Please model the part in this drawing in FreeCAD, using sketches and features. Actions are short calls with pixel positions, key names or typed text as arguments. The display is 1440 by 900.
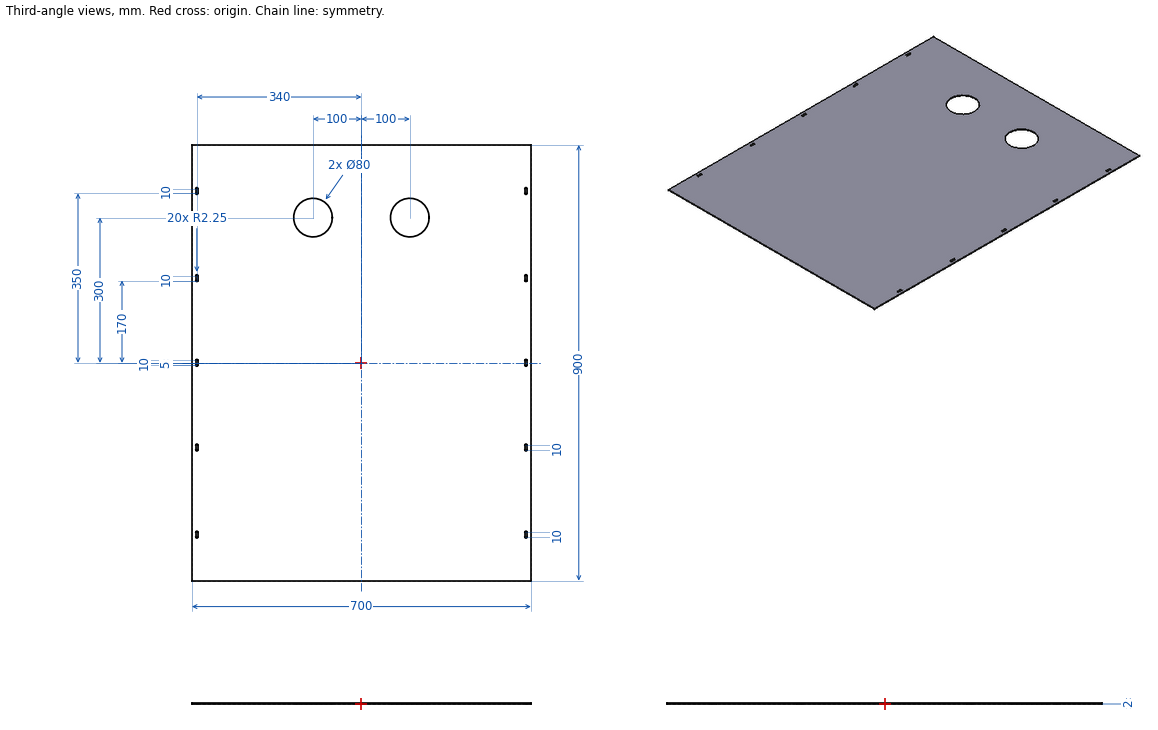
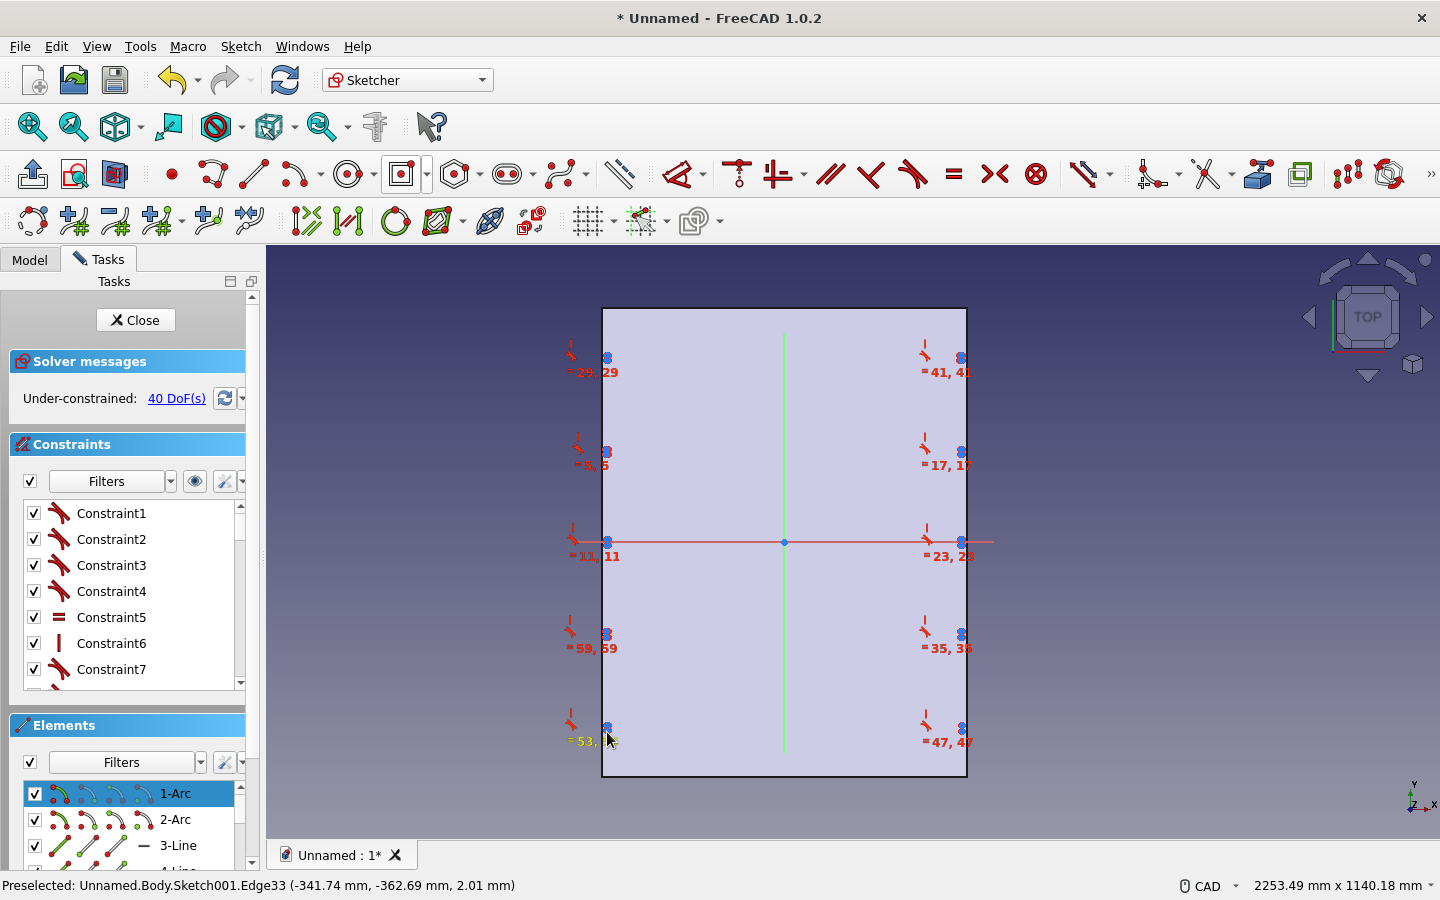
scroll(606, 639, up, 12)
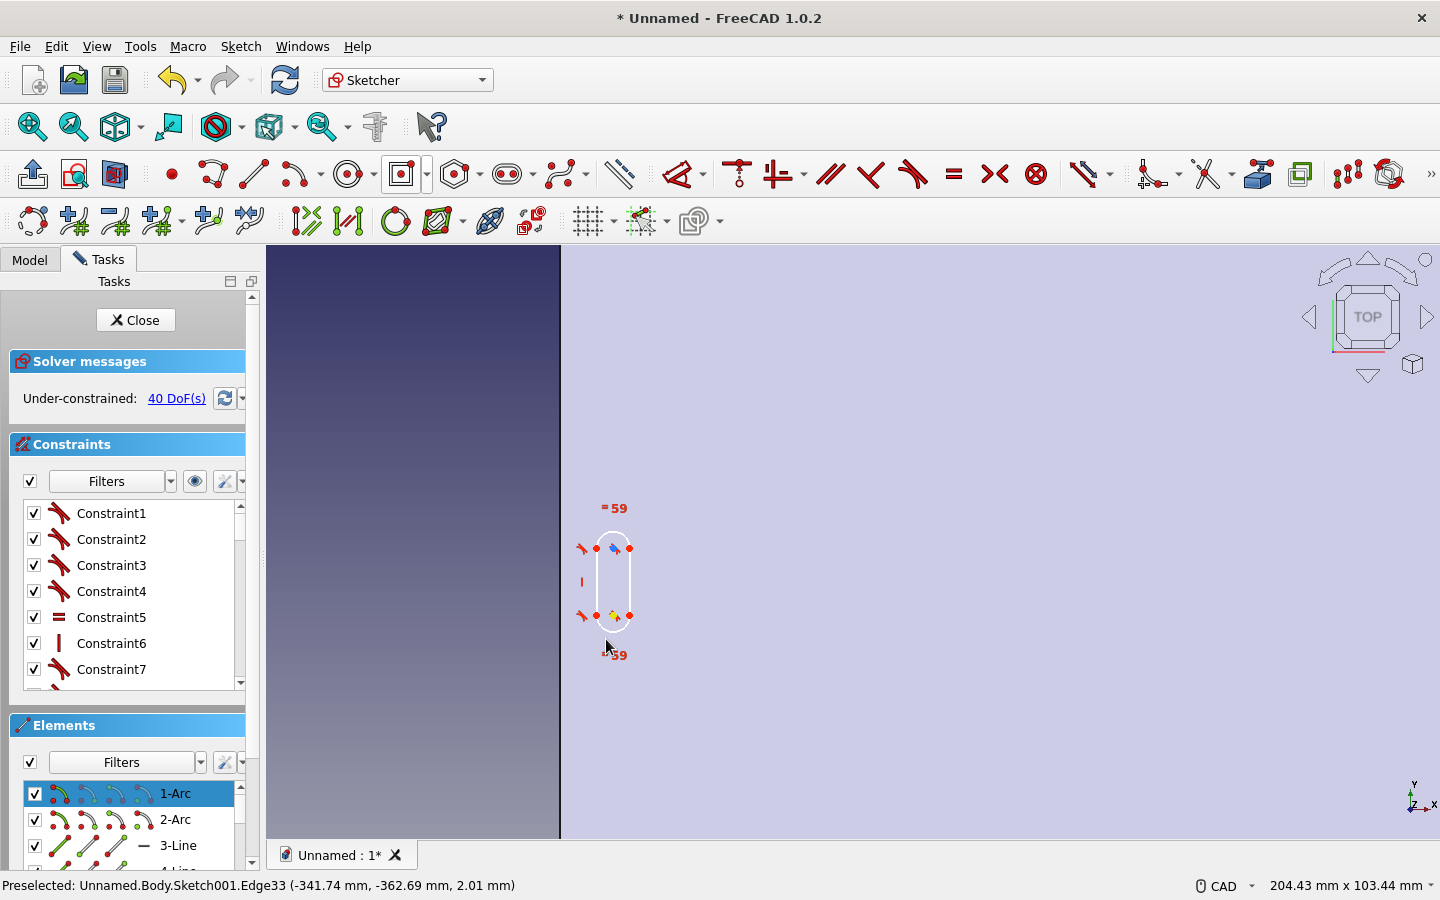
click(604, 629)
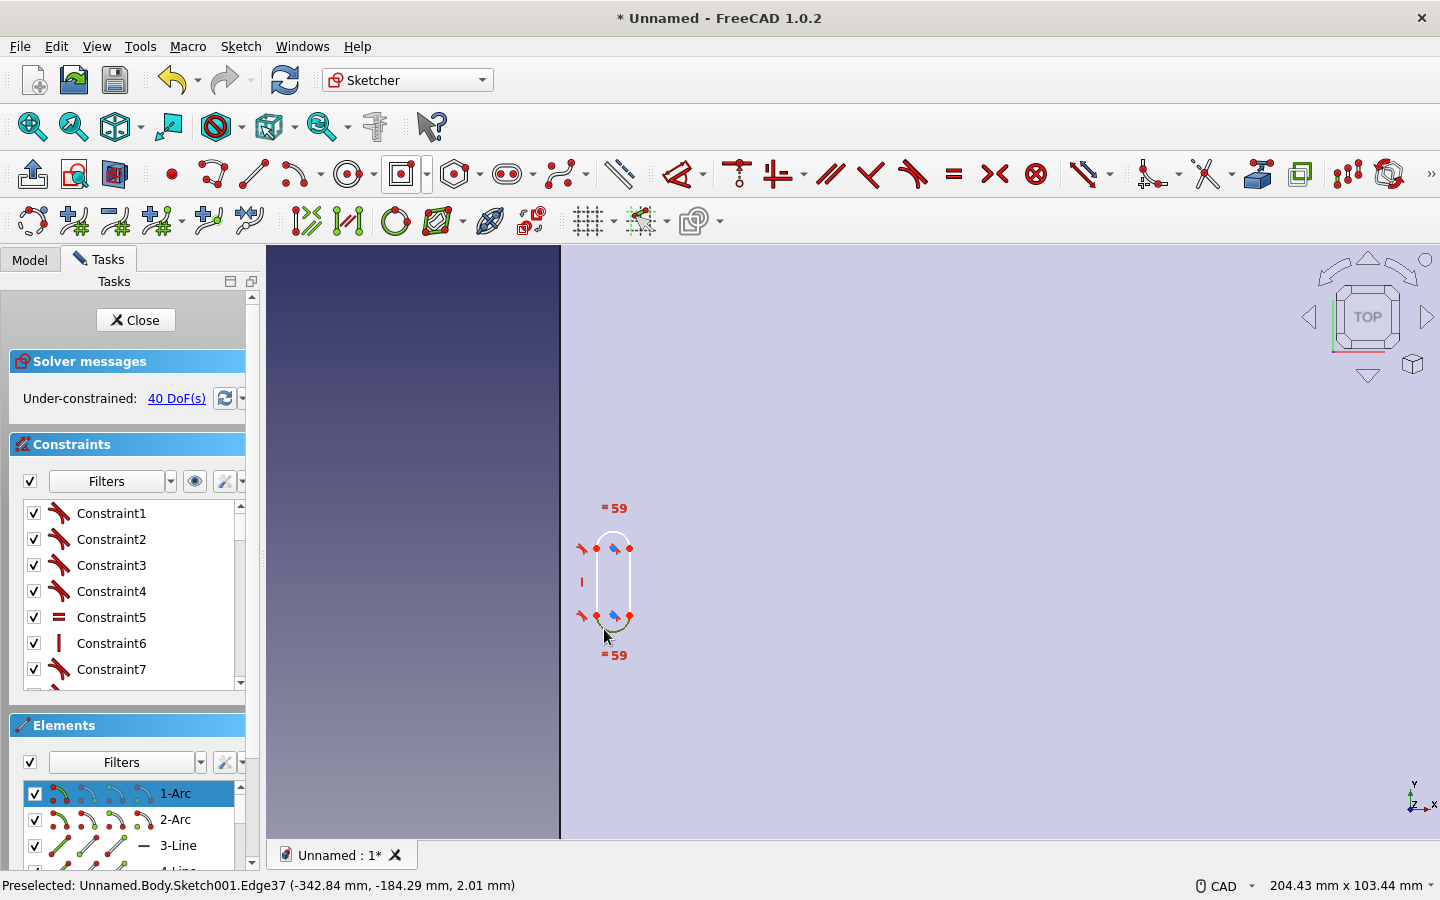
key(e)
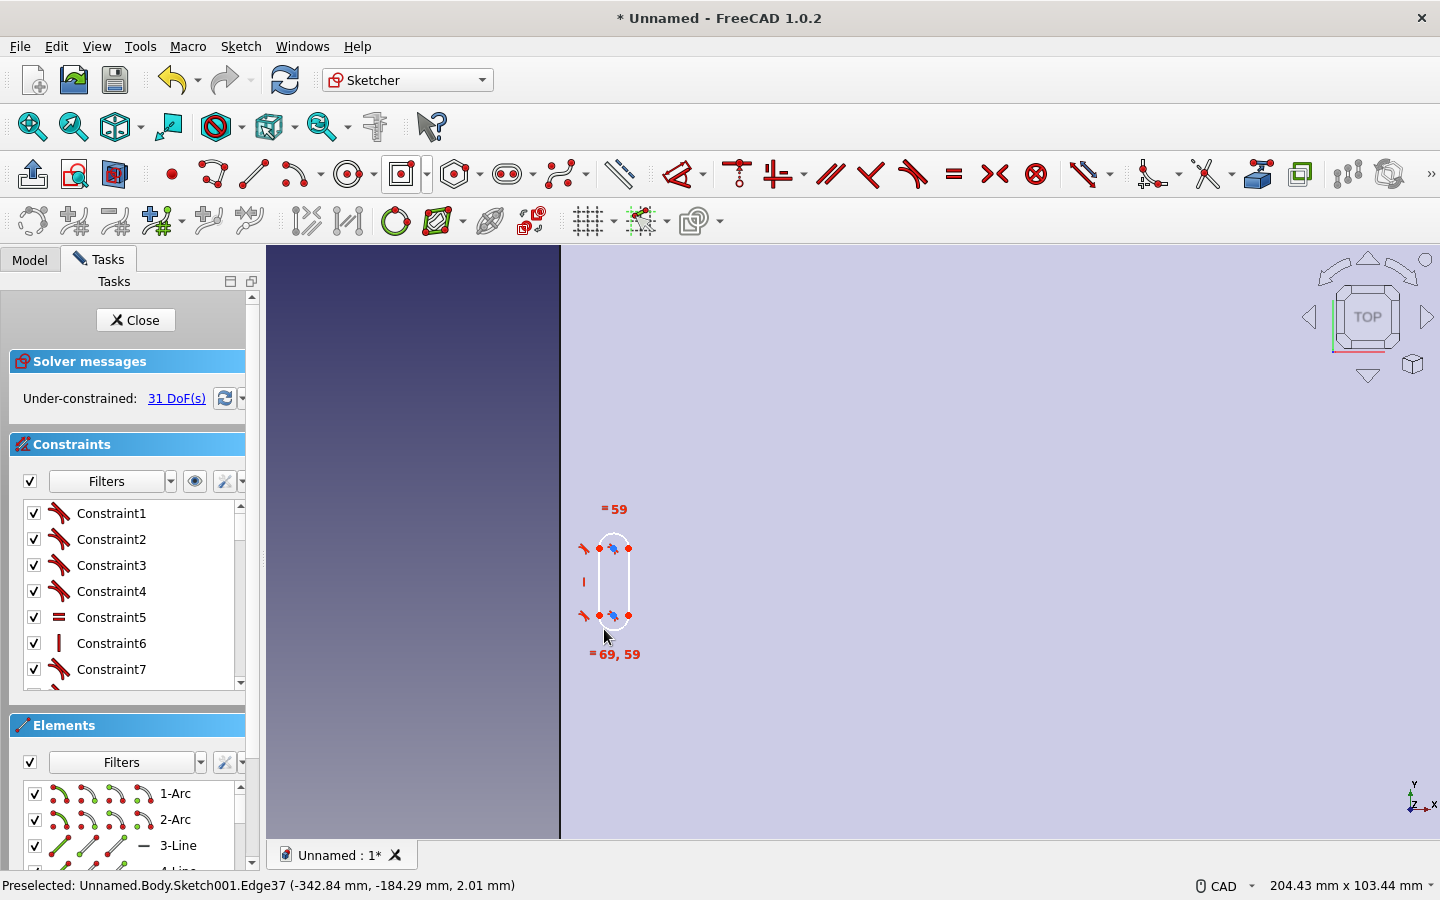
scroll(606, 639, down, 12)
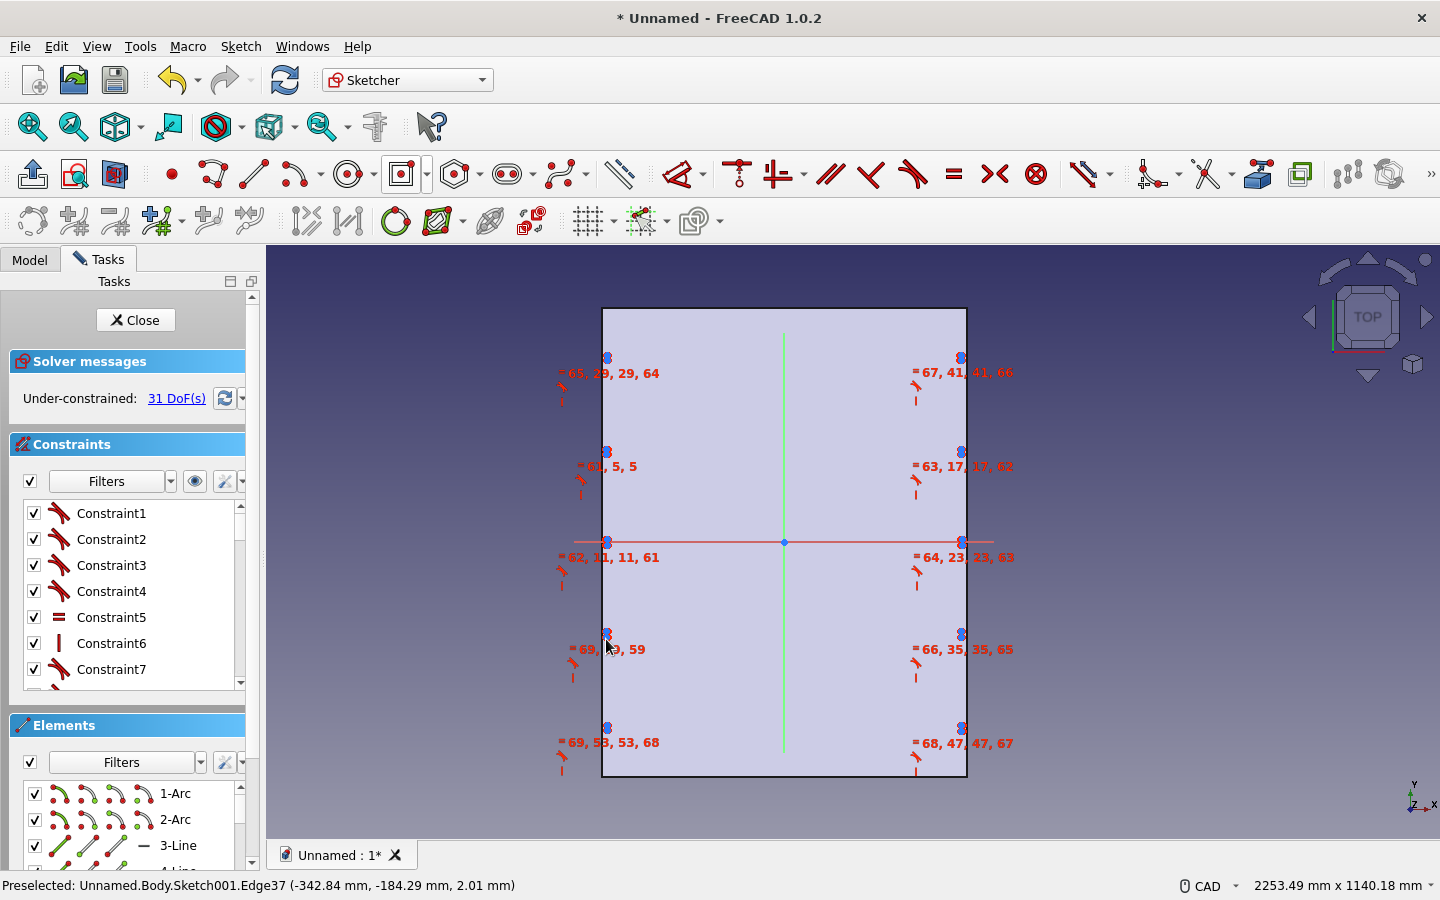
scroll(607, 454, up, 12)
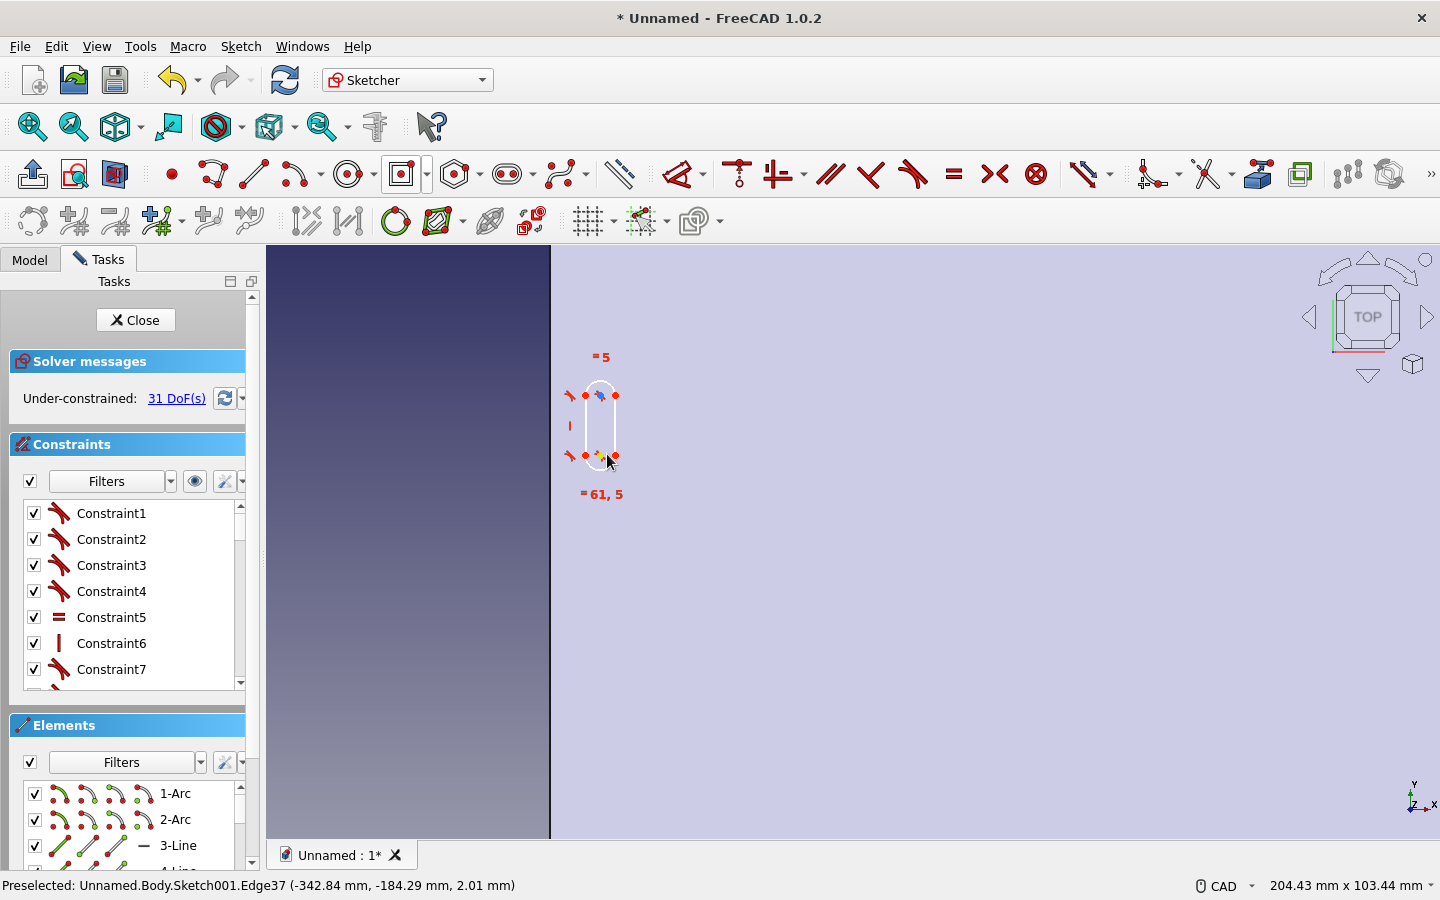
click(600, 456)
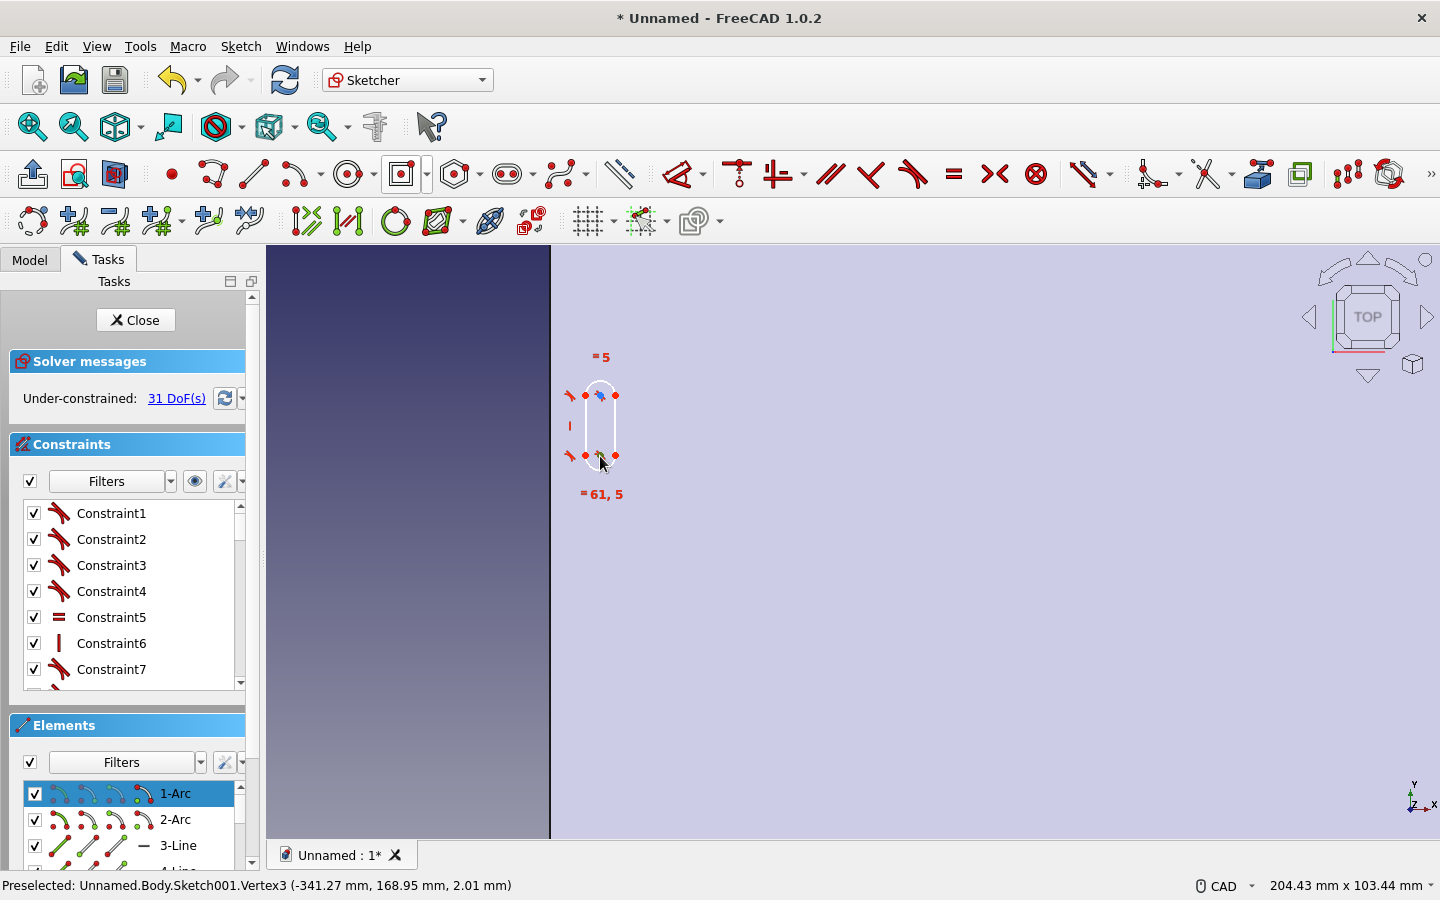
scroll(607, 454, down, 12)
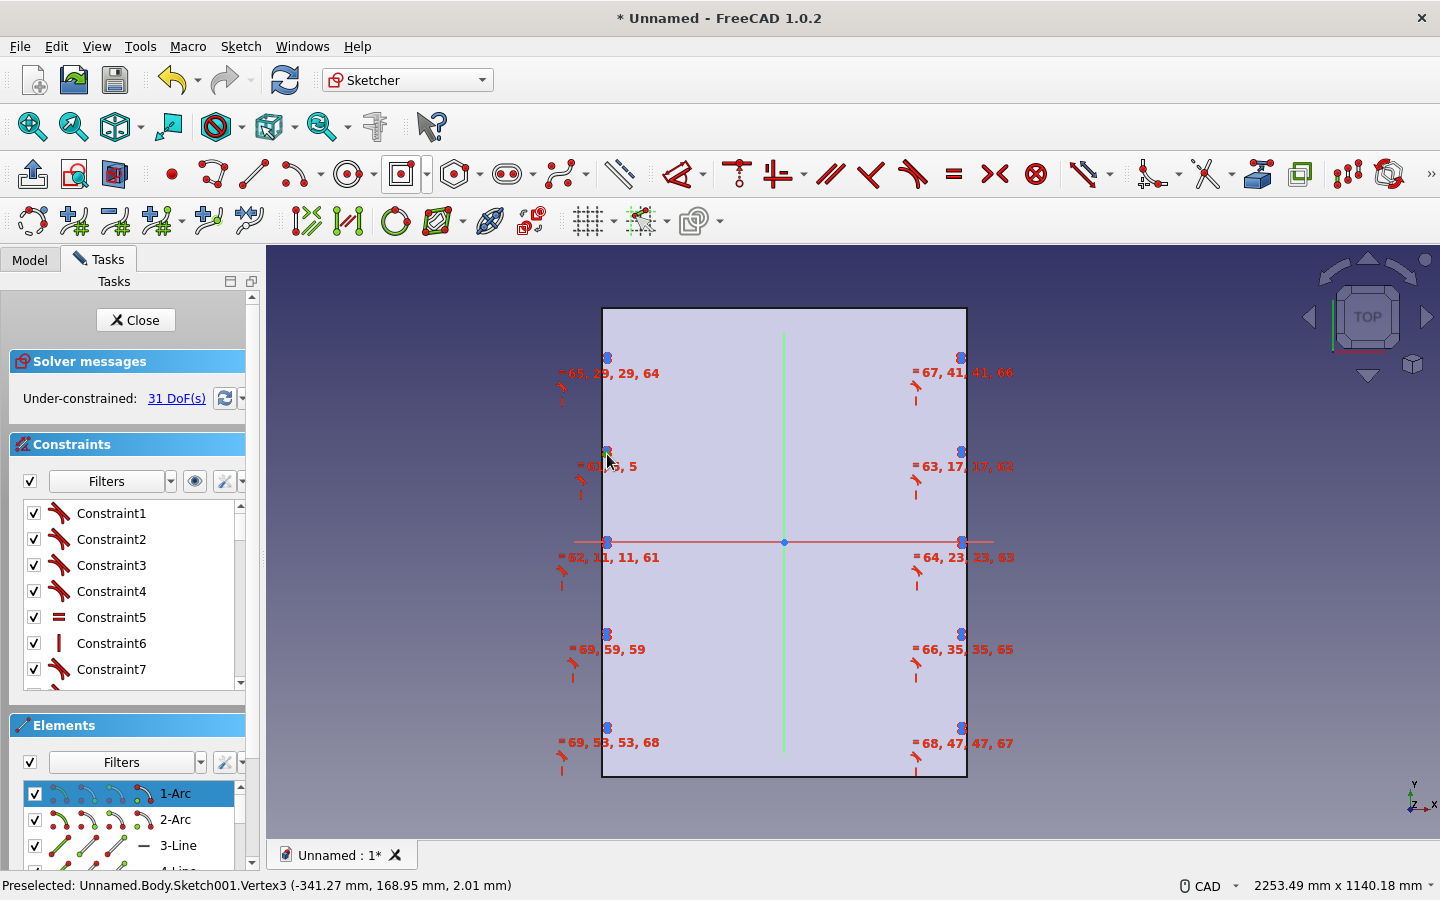
scroll(961, 455, up, 12)